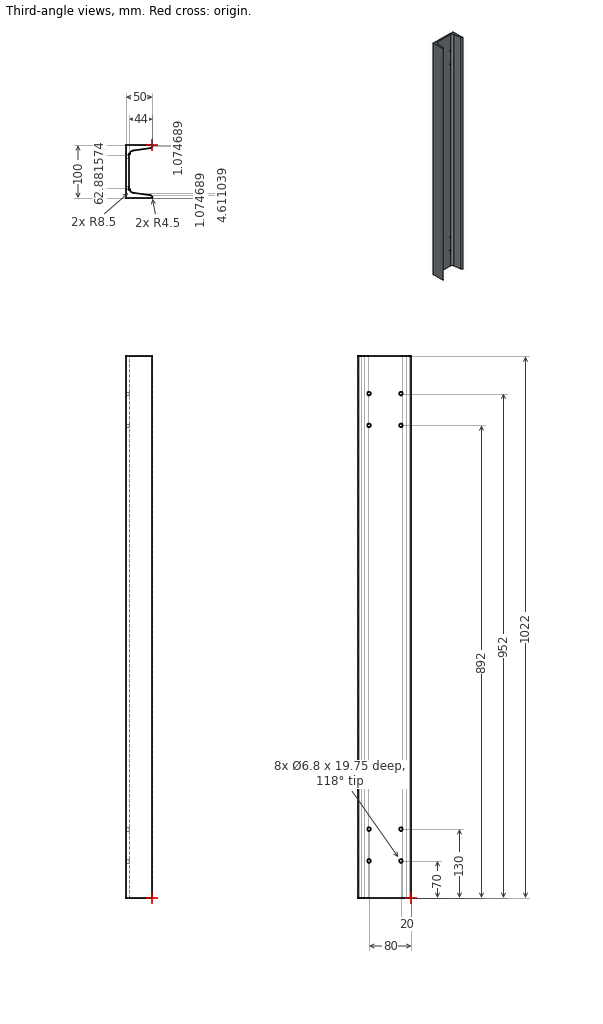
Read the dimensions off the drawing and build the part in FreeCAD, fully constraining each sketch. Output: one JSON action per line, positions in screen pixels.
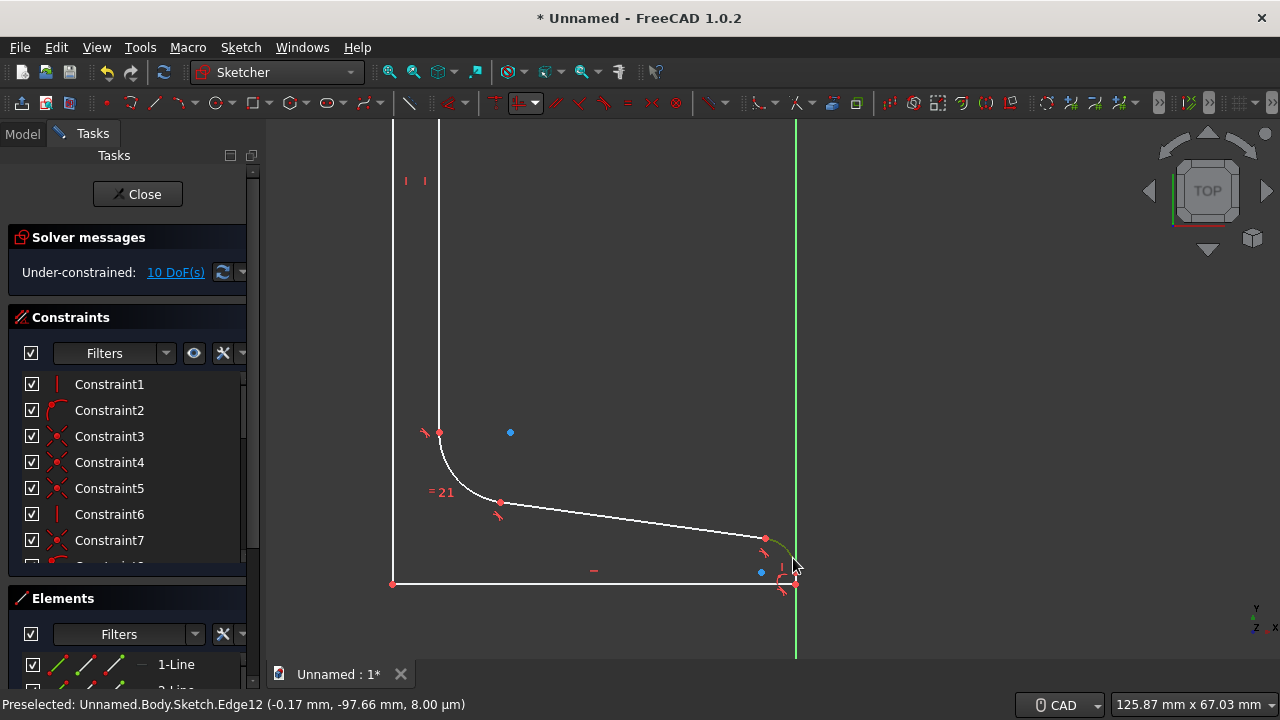
{"action": "left_click", "coordinate": [628, 104]}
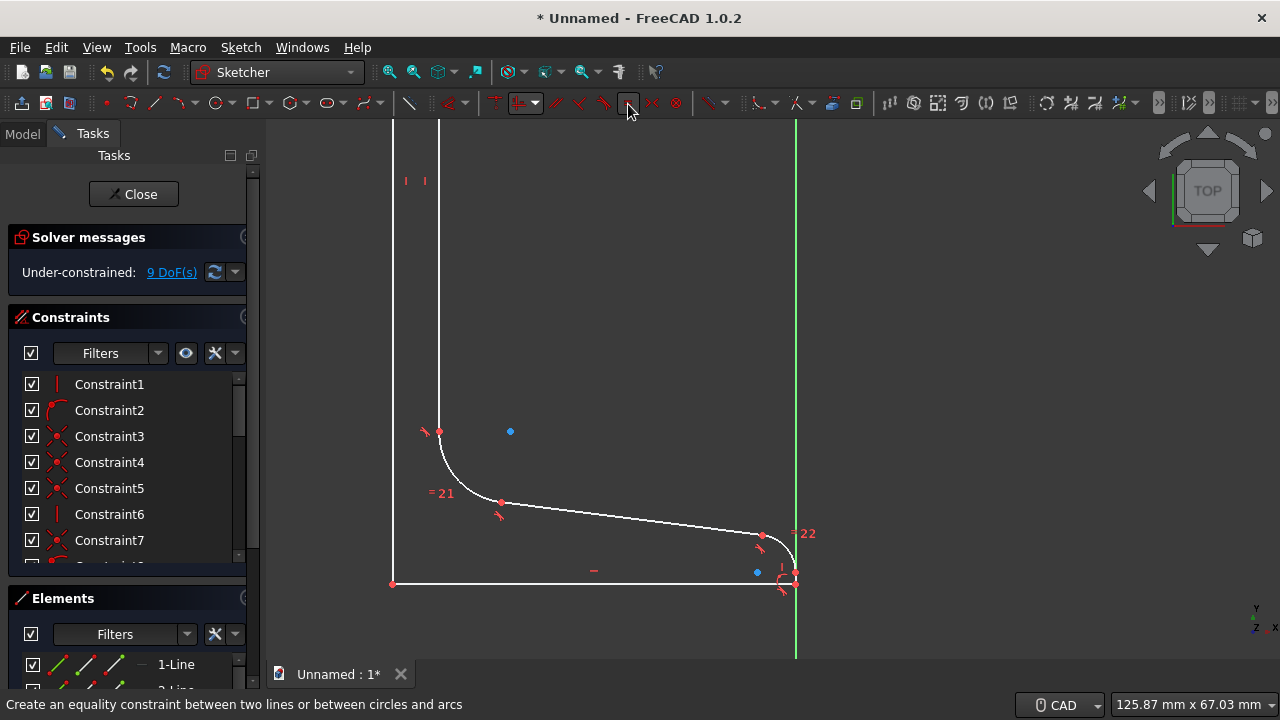
{"action": "left_click", "coordinate": [448, 104]}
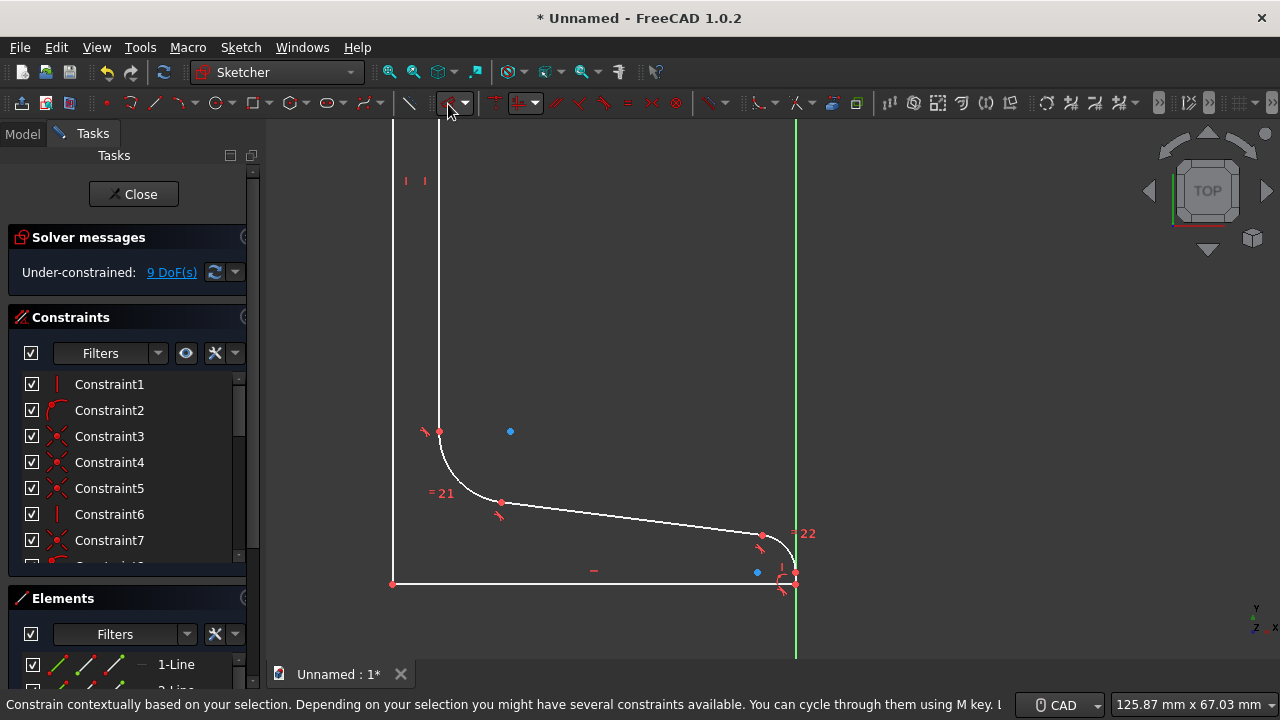
{"action": "left_click", "coordinate": [446, 462]}
{"action": "left_click", "coordinate": [417, 476]}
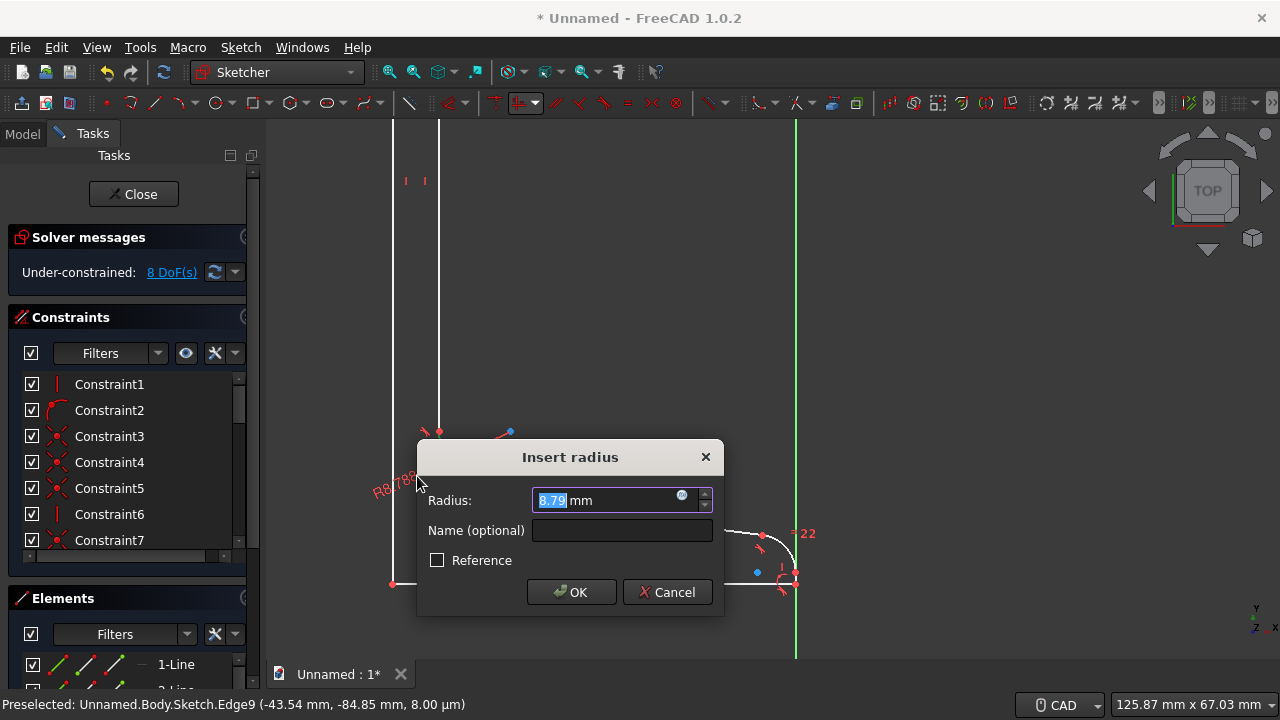
{"action": "type", "text": "8.5"}
{"action": "key", "text": "Return"}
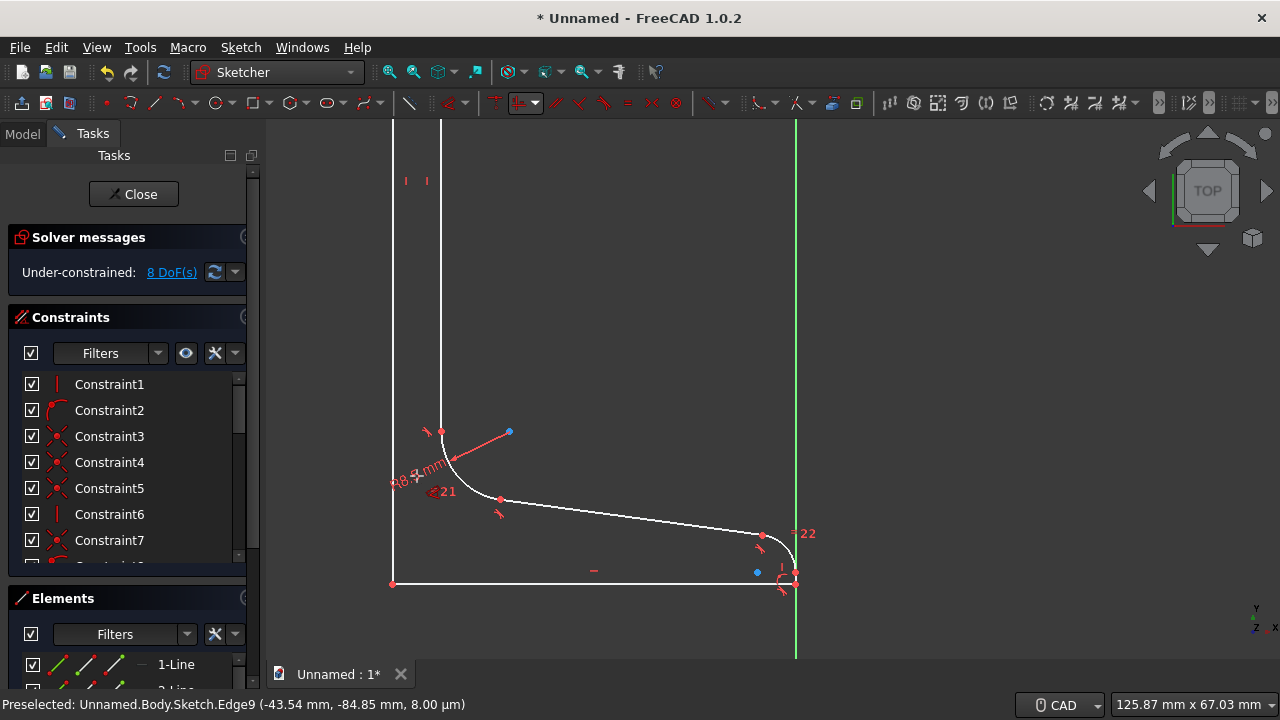
{"action": "scroll", "coordinate": [794, 560], "scroll_direction": "down", "scroll_amount": 4}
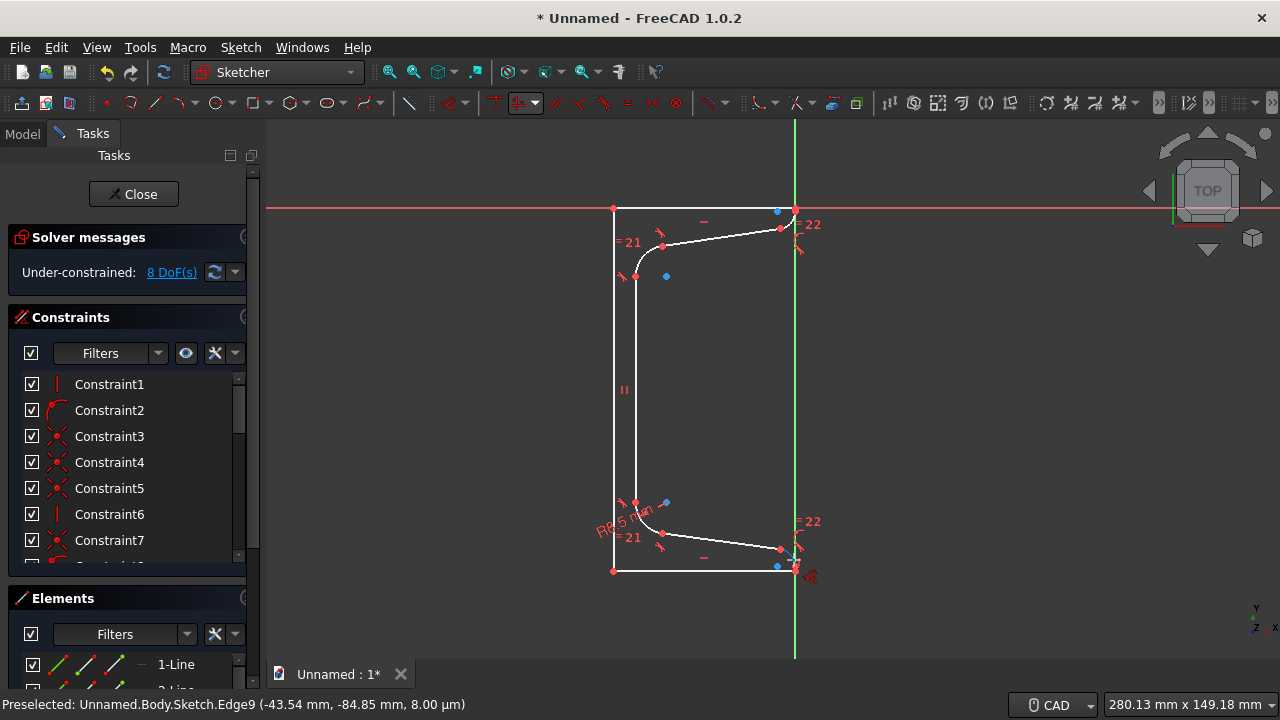
{"action": "scroll", "coordinate": [787, 226], "scroll_direction": "up", "scroll_amount": 5}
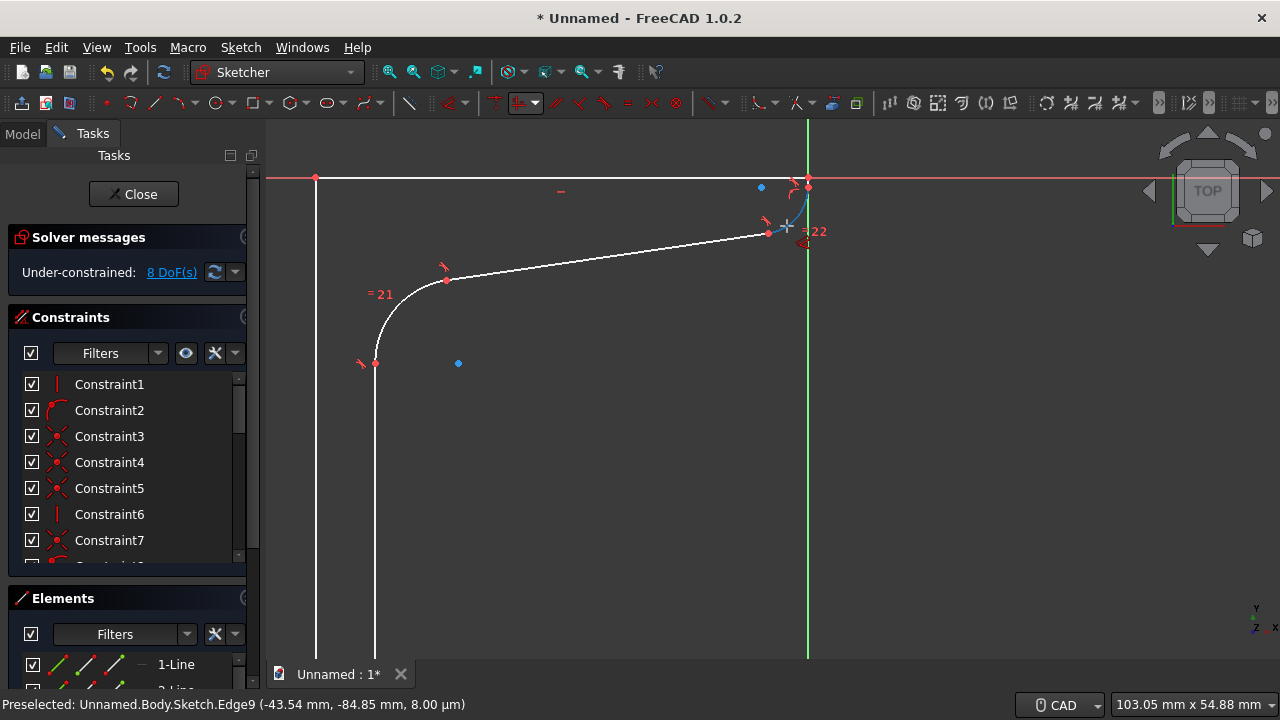
{"action": "left_click", "coordinate": [787, 227]}
{"action": "left_click", "coordinate": [767, 266]}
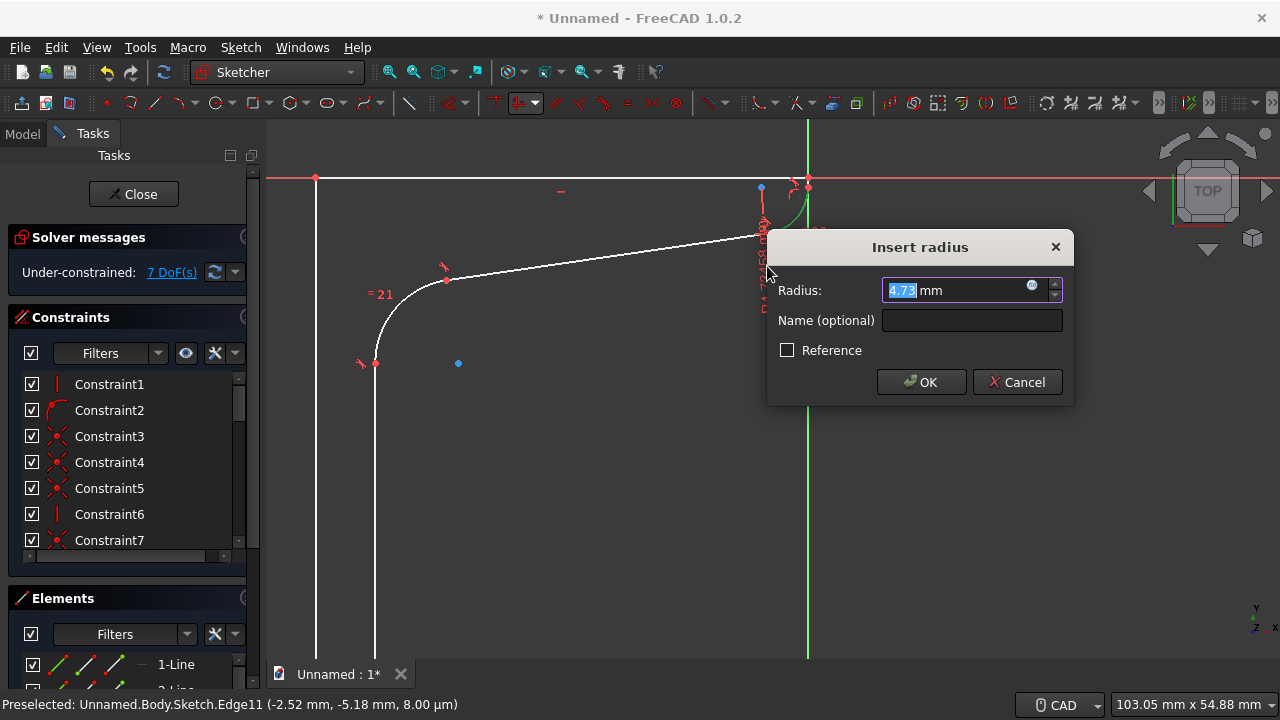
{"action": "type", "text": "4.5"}
{"action": "key", "text": "Return"}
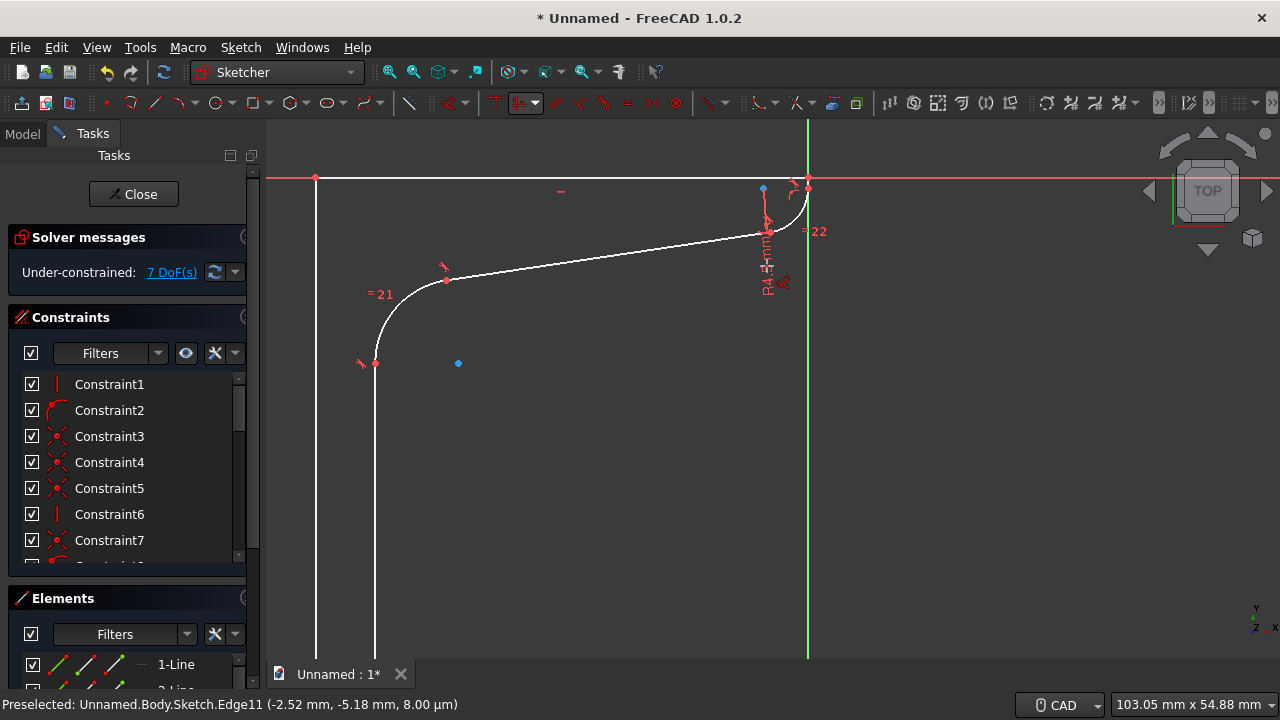
{"action": "left_click", "coordinate": [660, 178]}
{"action": "left_click", "coordinate": [562, 212]}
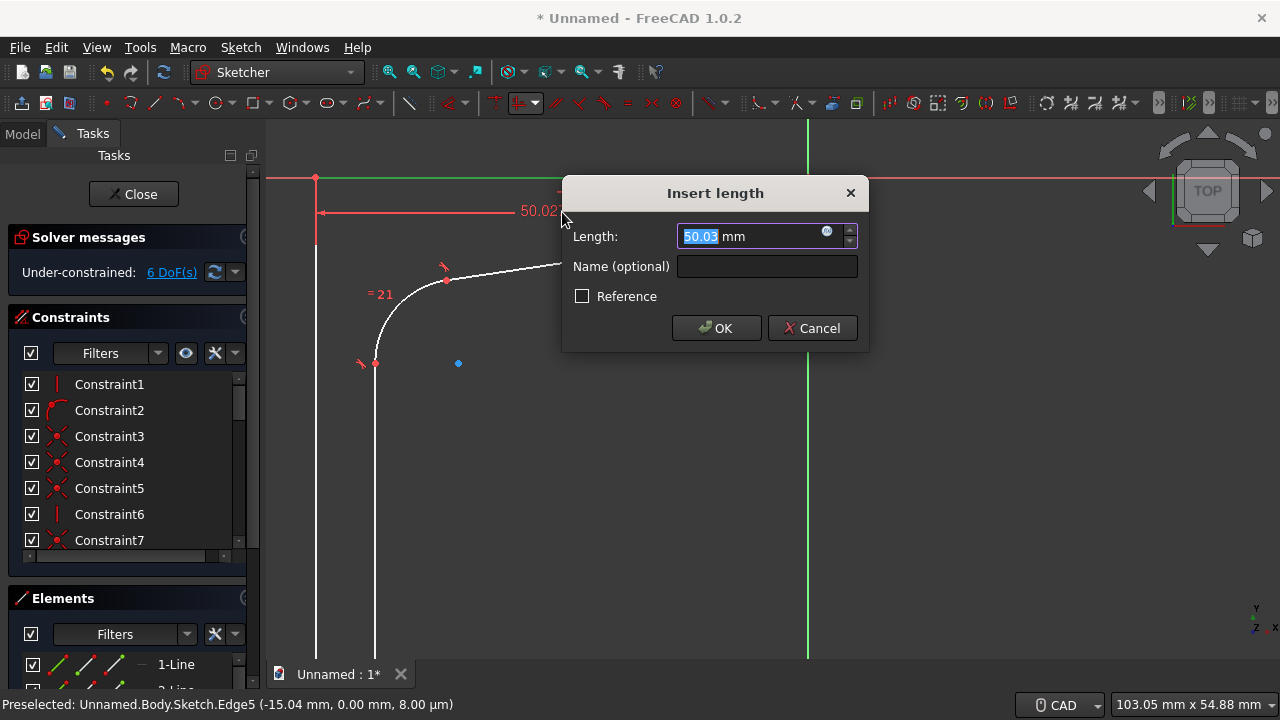
{"action": "type", "text": "50"}
{"action": "key", "text": "Return"}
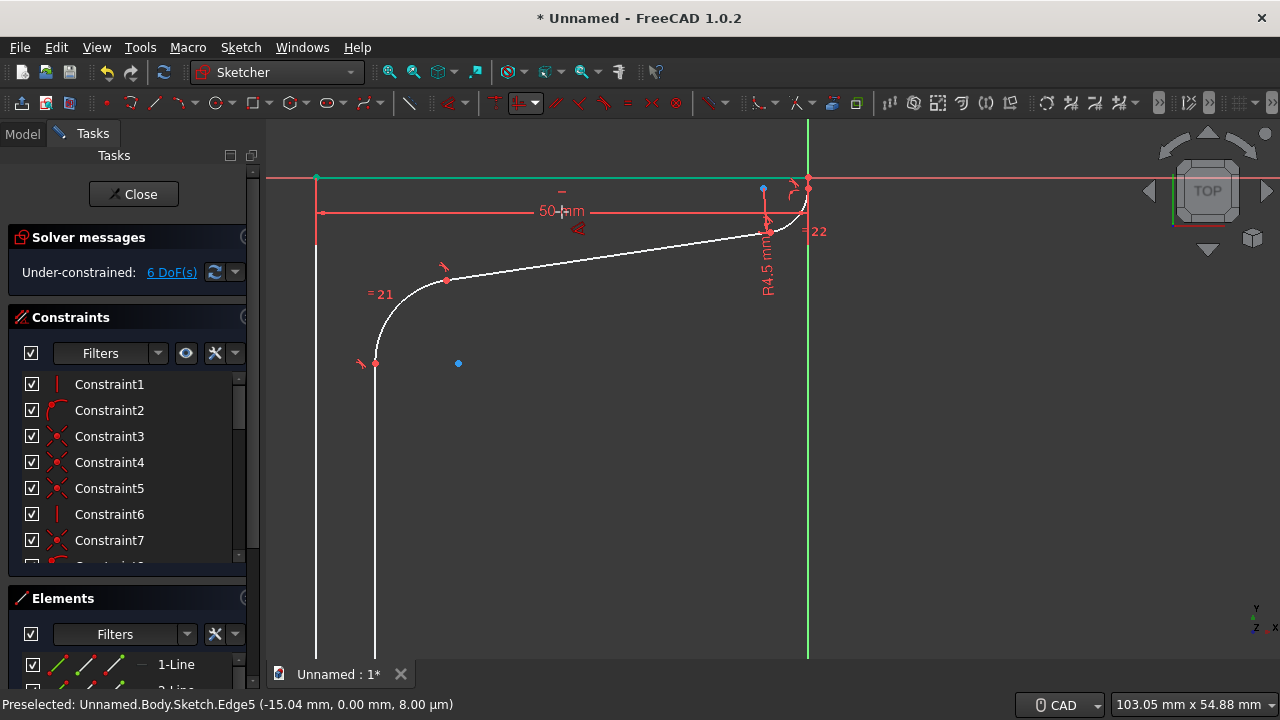
{"action": "left_click", "coordinate": [316, 474]}
{"action": "left_click", "coordinate": [350, 404]}